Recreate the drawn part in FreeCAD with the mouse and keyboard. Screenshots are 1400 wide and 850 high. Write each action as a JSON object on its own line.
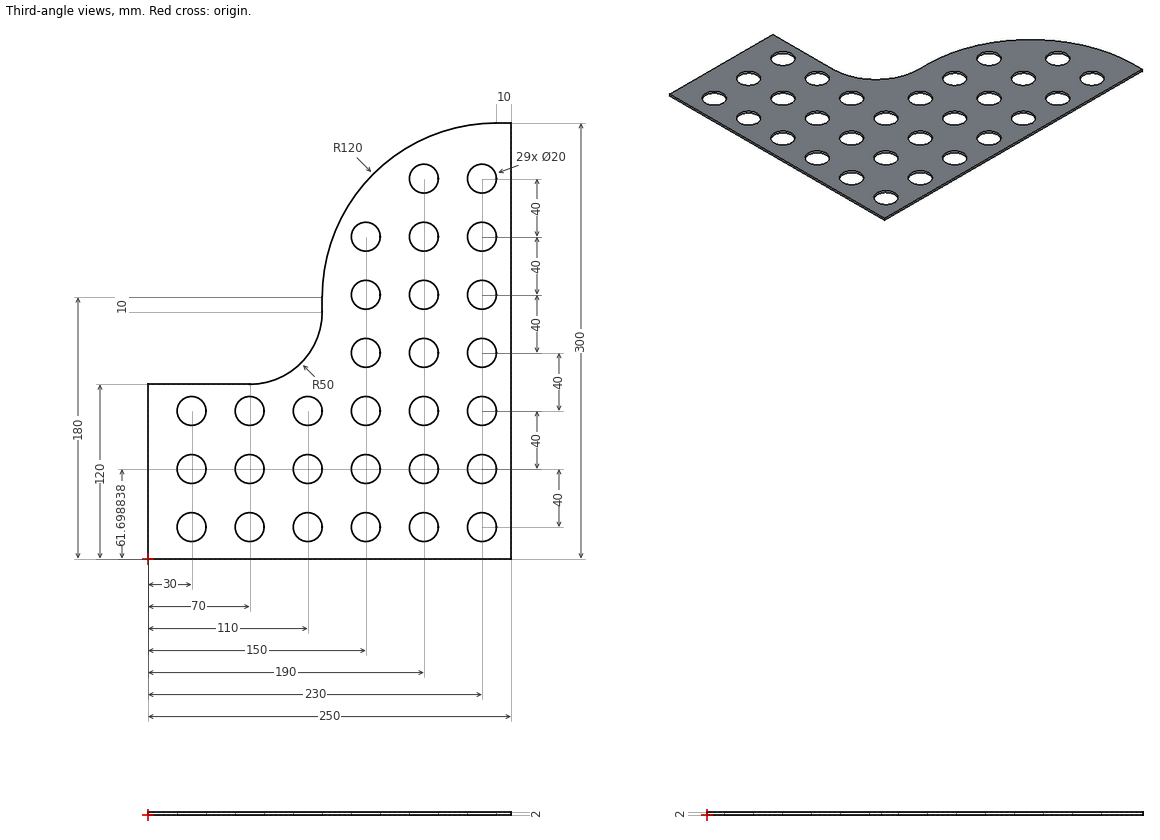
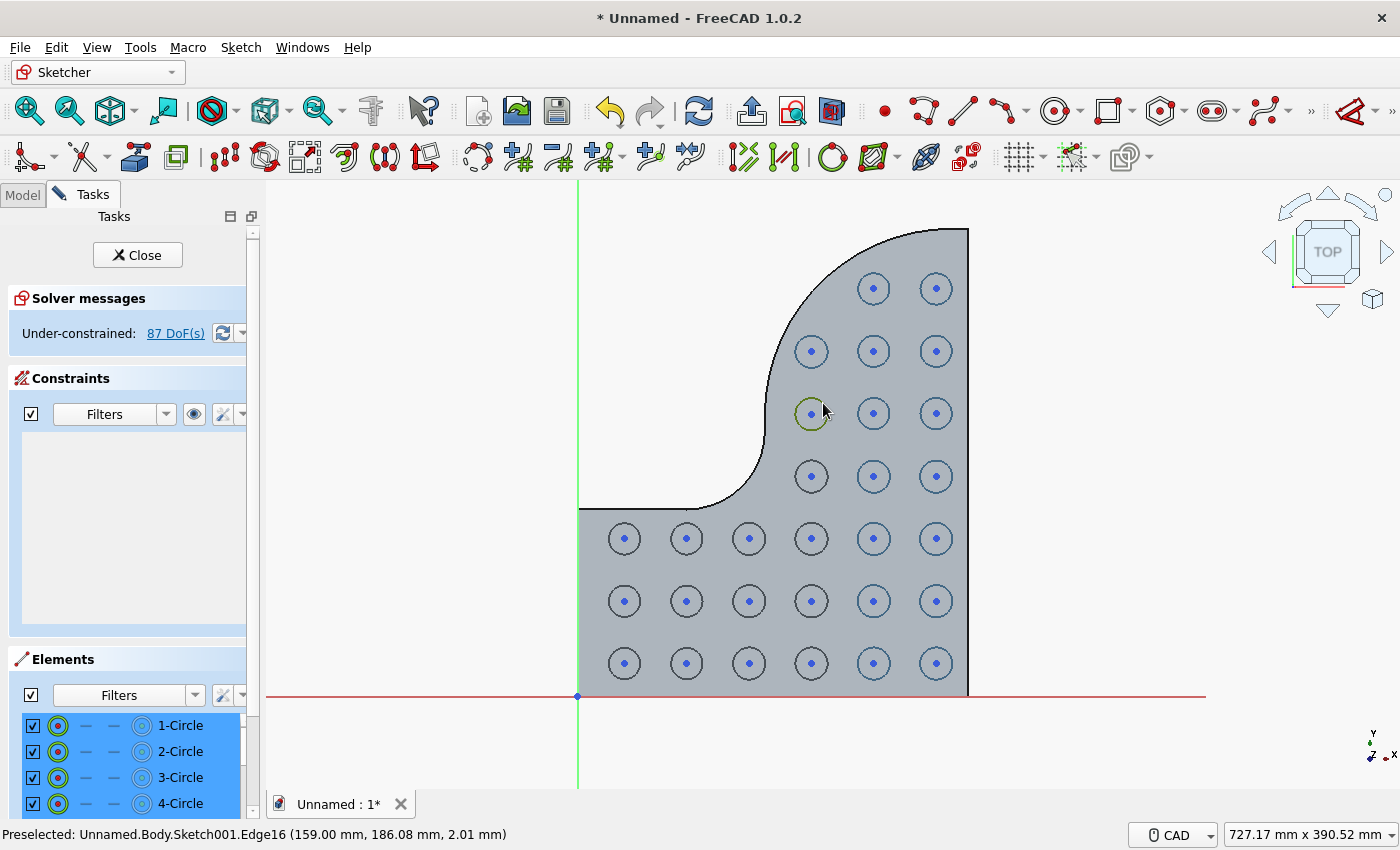
{"action": "left_click", "coordinate": [823, 465]}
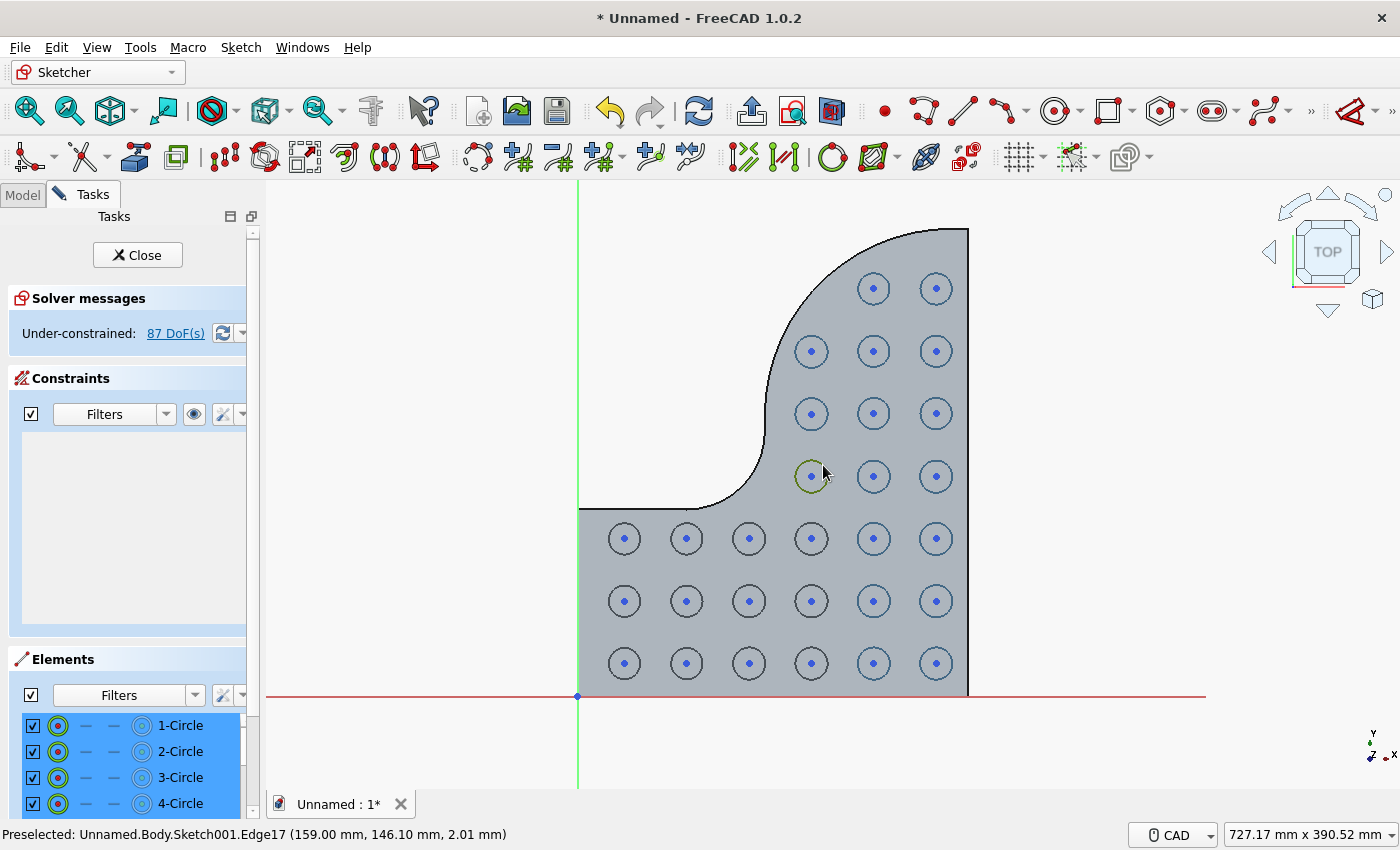
{"action": "left_click", "coordinate": [823, 527]}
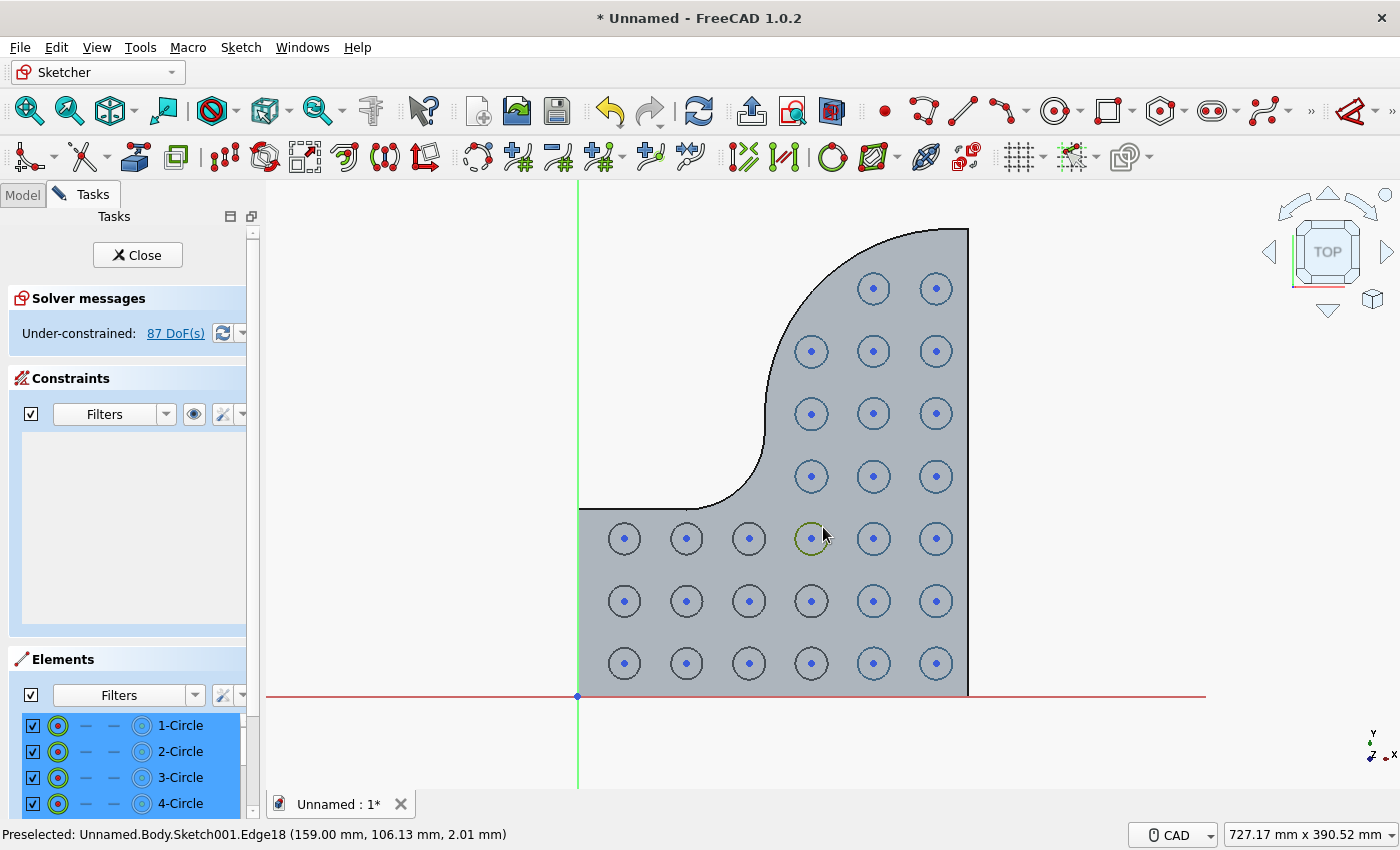
{"action": "left_click", "coordinate": [823, 590]}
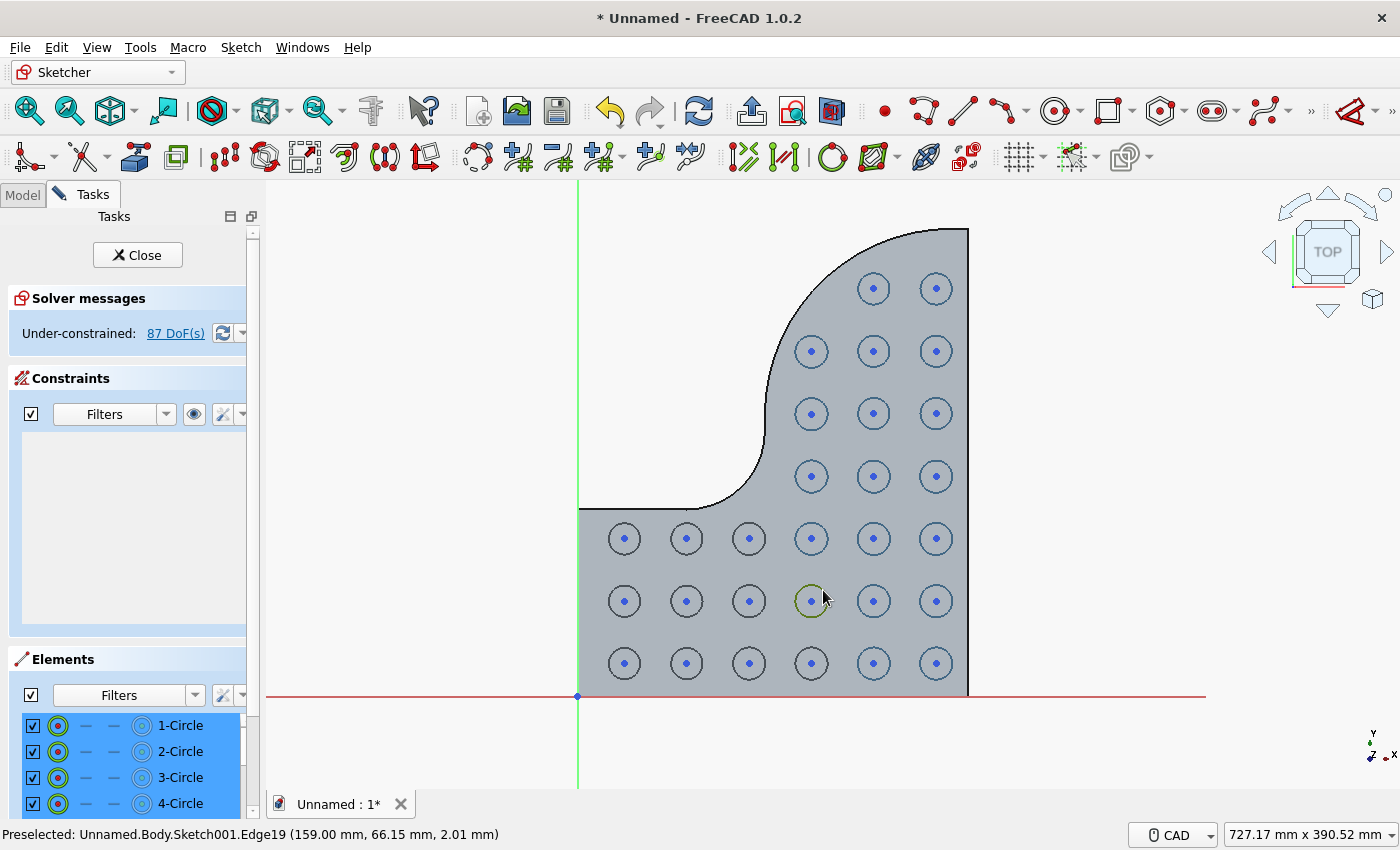
{"action": "left_click", "coordinate": [823, 652]}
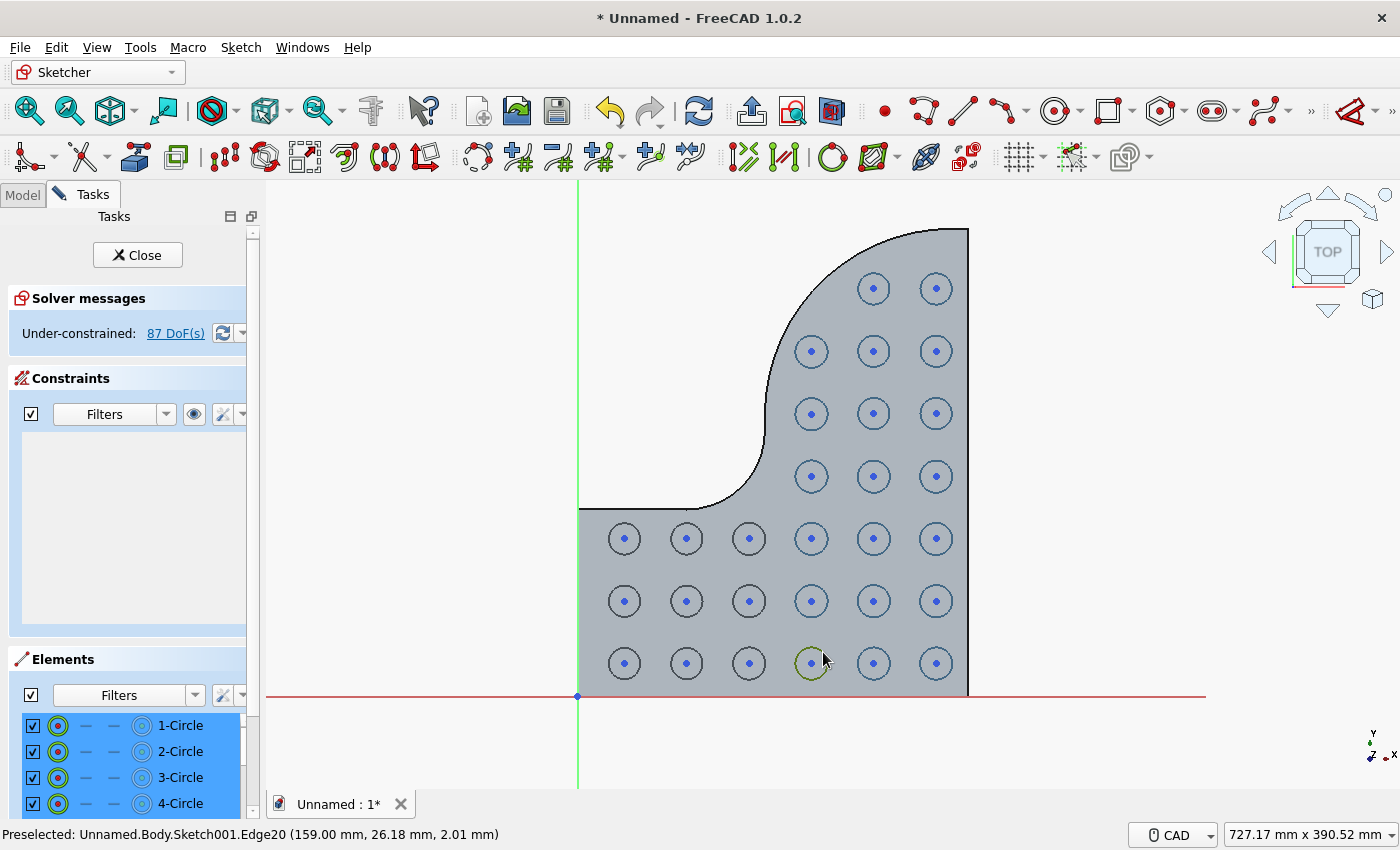
{"action": "left_click", "coordinate": [761, 527]}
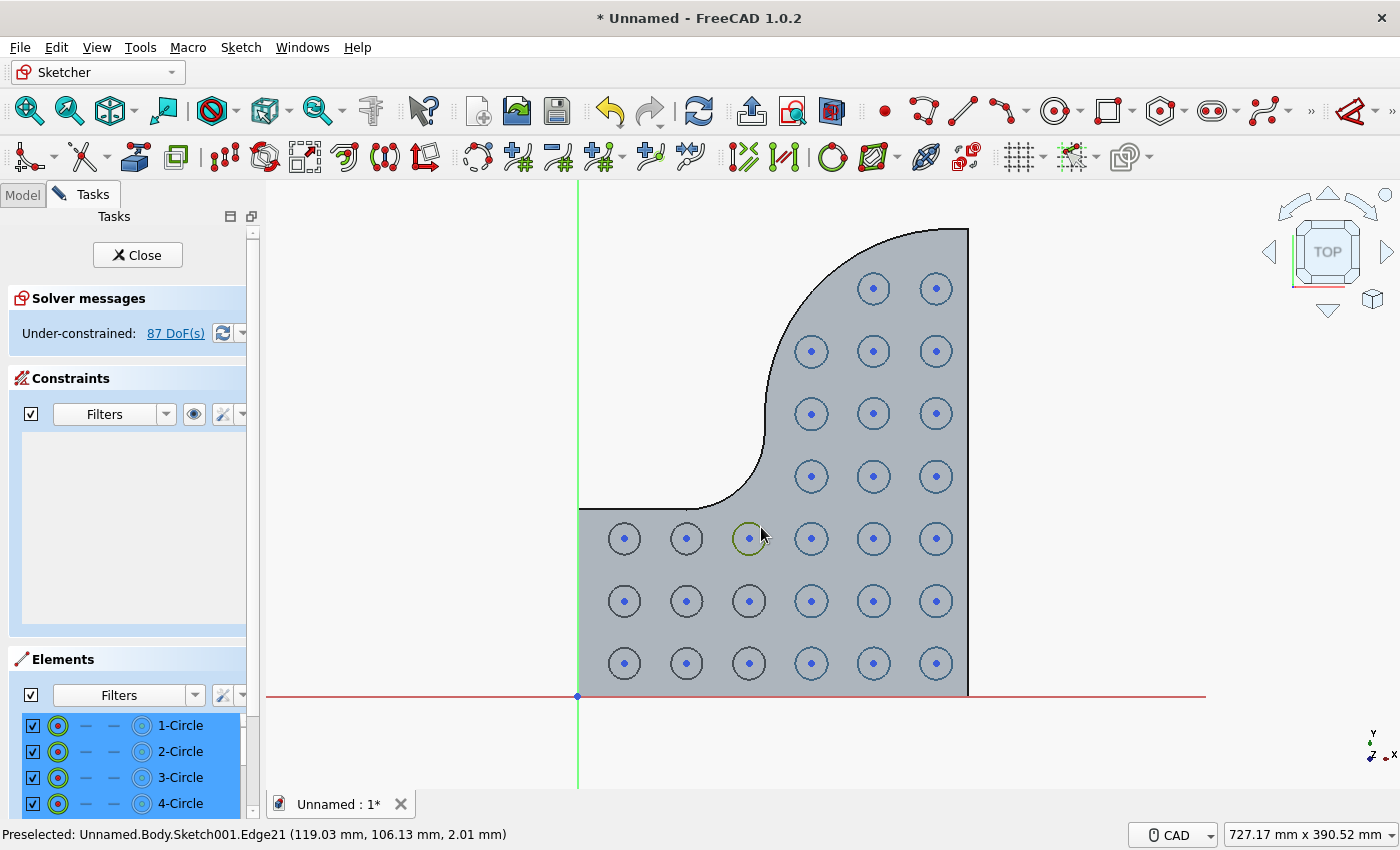
{"action": "left_click", "coordinate": [698, 528]}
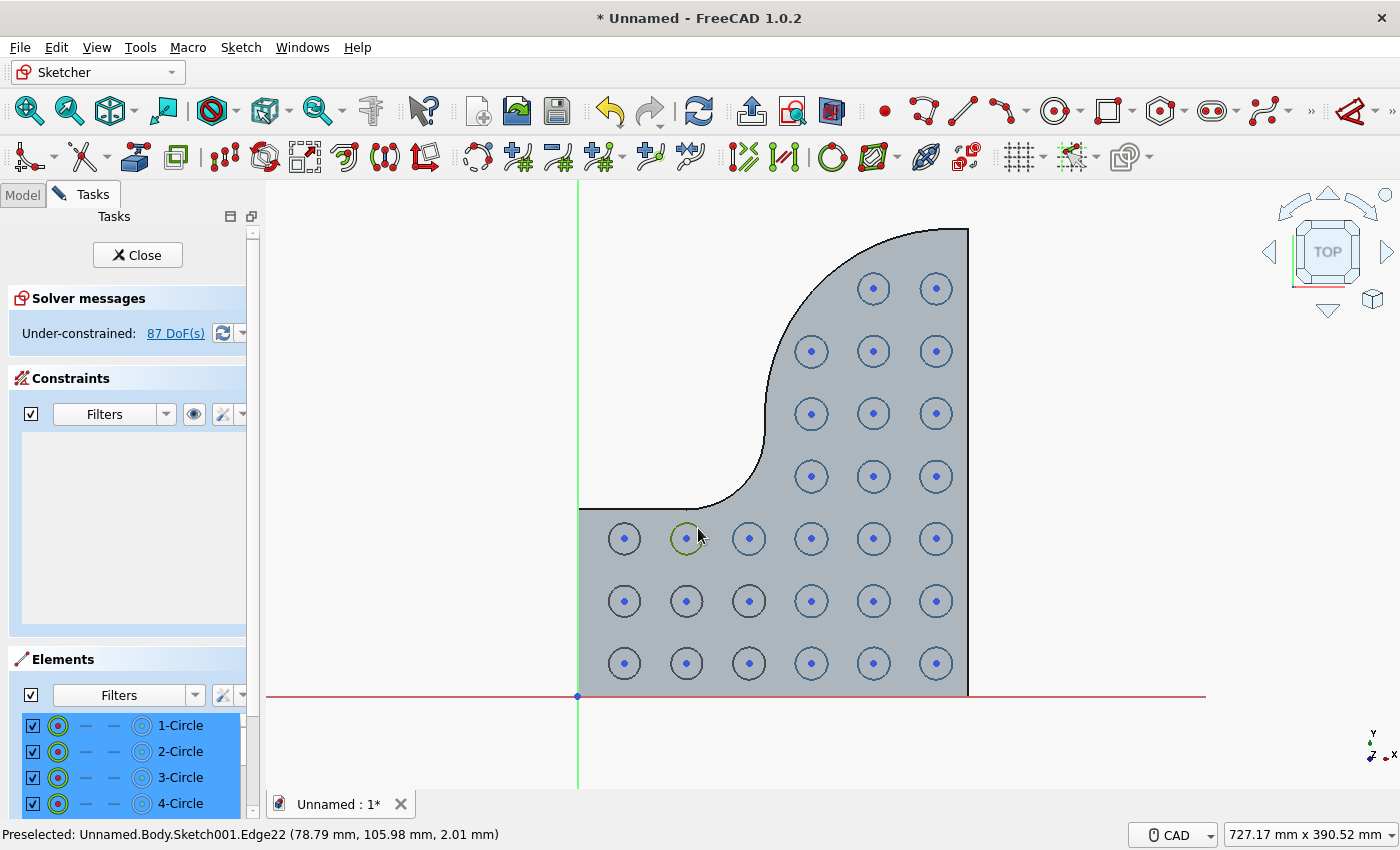
{"action": "left_click", "coordinate": [636, 528]}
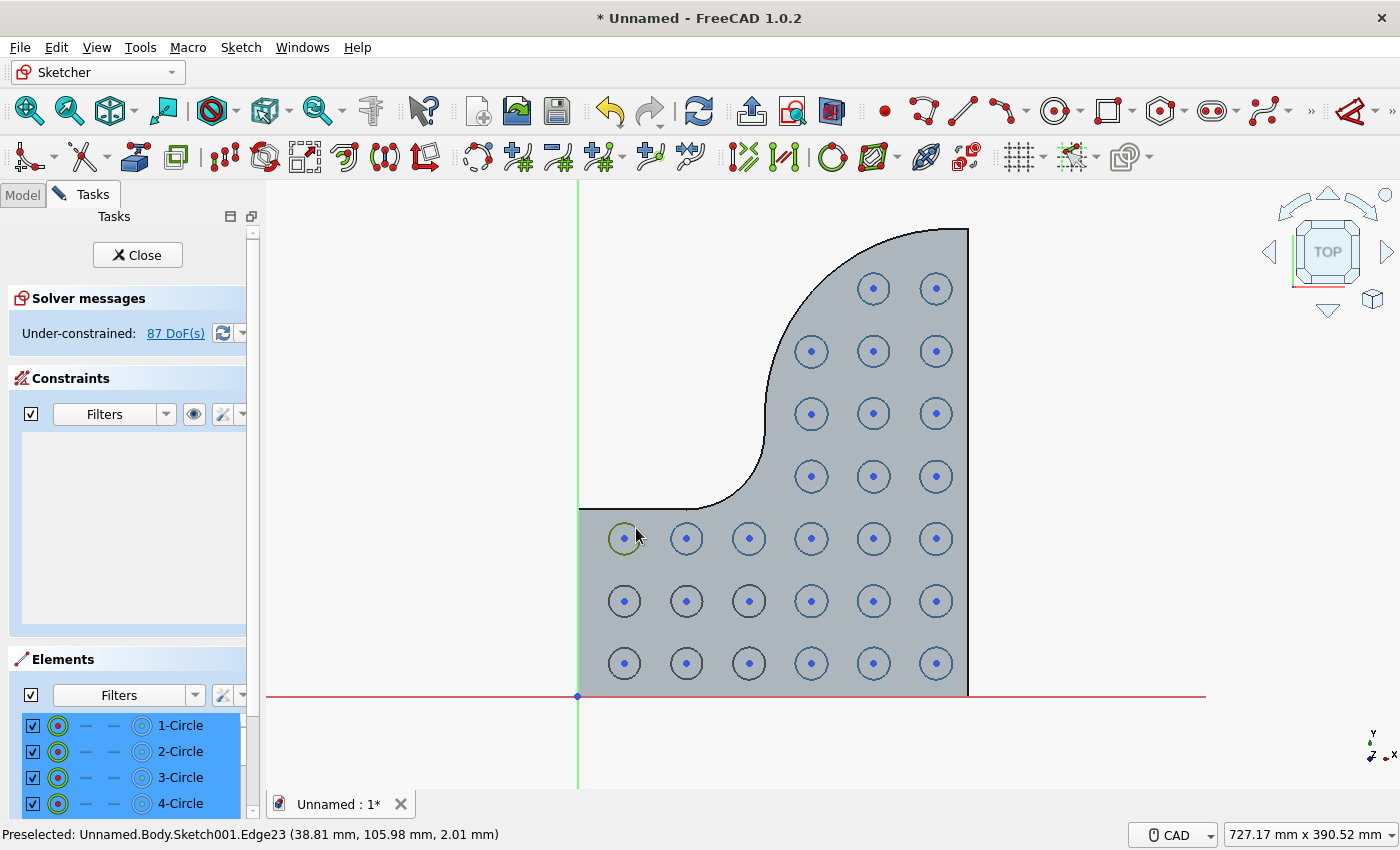
{"action": "left_click", "coordinate": [761, 590]}